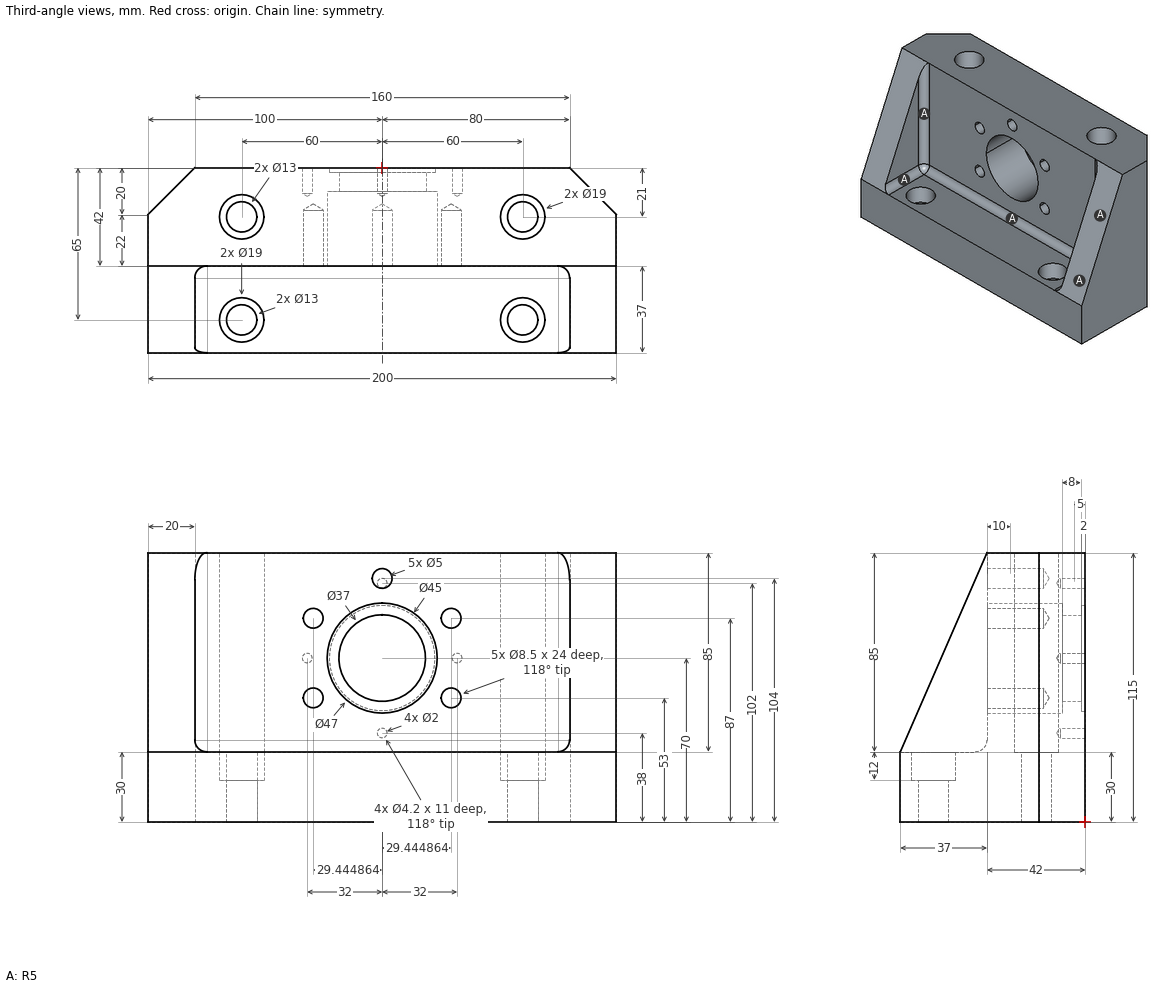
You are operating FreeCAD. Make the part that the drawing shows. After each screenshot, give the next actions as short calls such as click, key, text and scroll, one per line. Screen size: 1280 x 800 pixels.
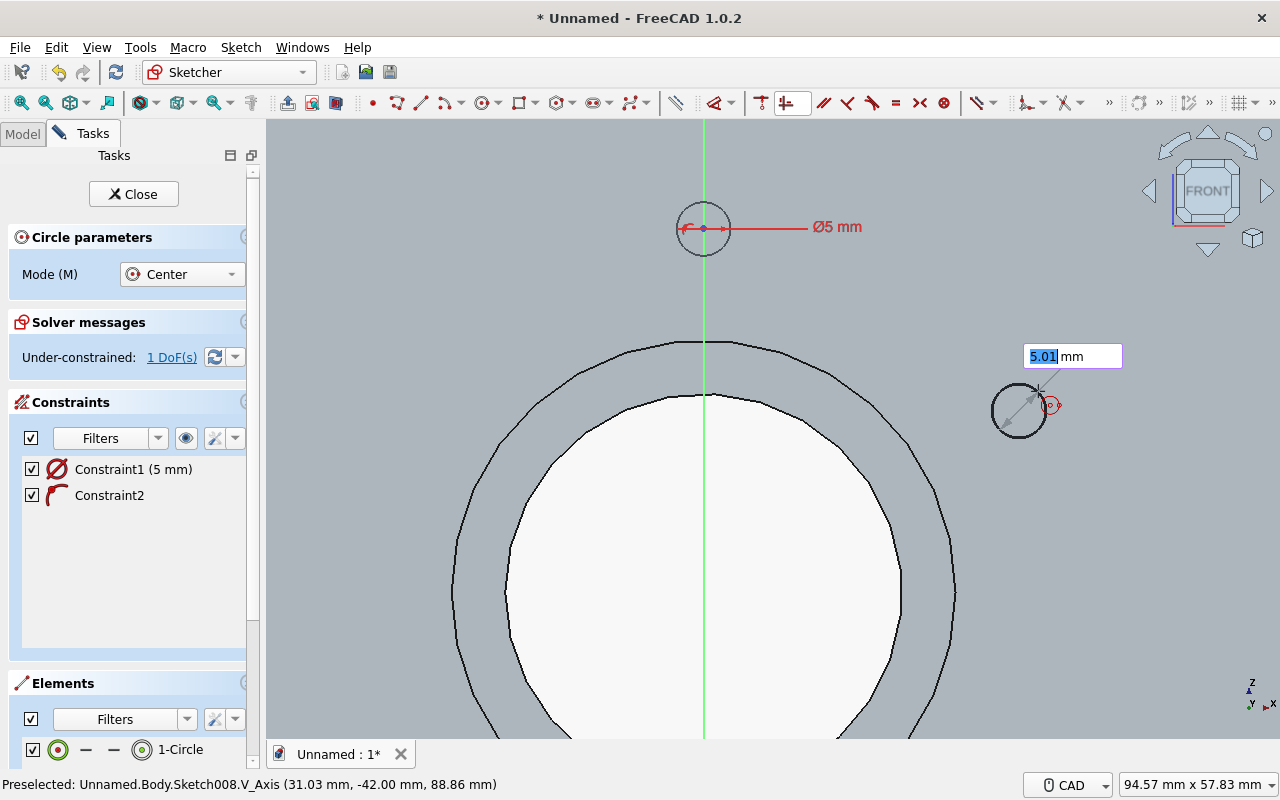
text(5)
key(Return)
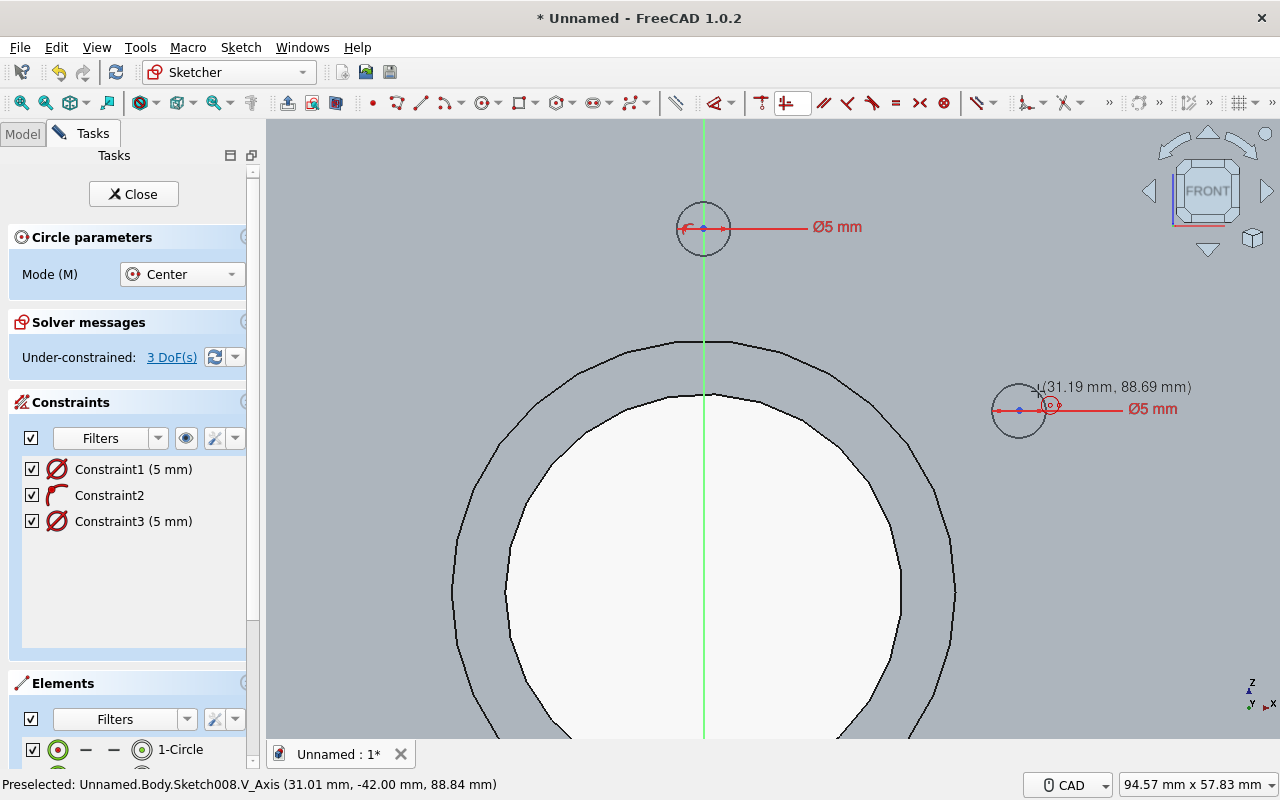
scroll(705, 229, down, 5)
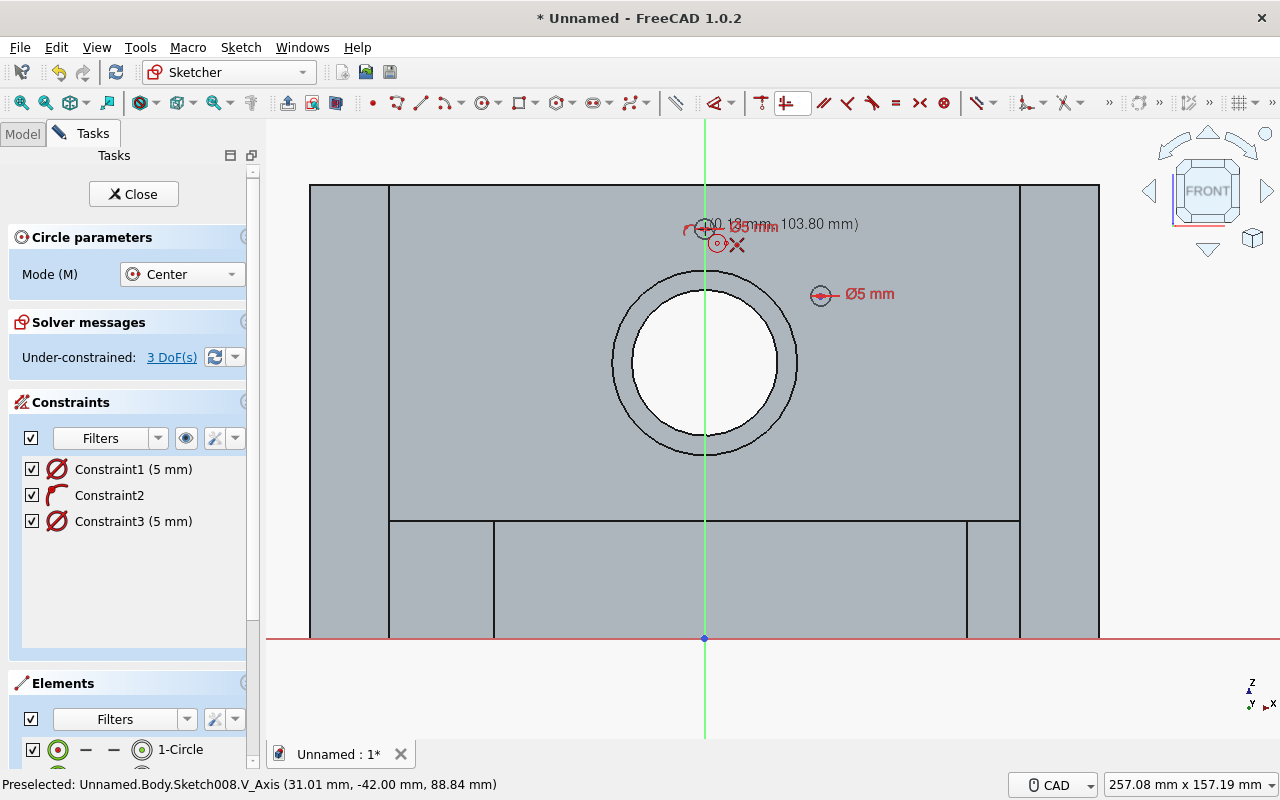
scroll(821, 430, up, 5)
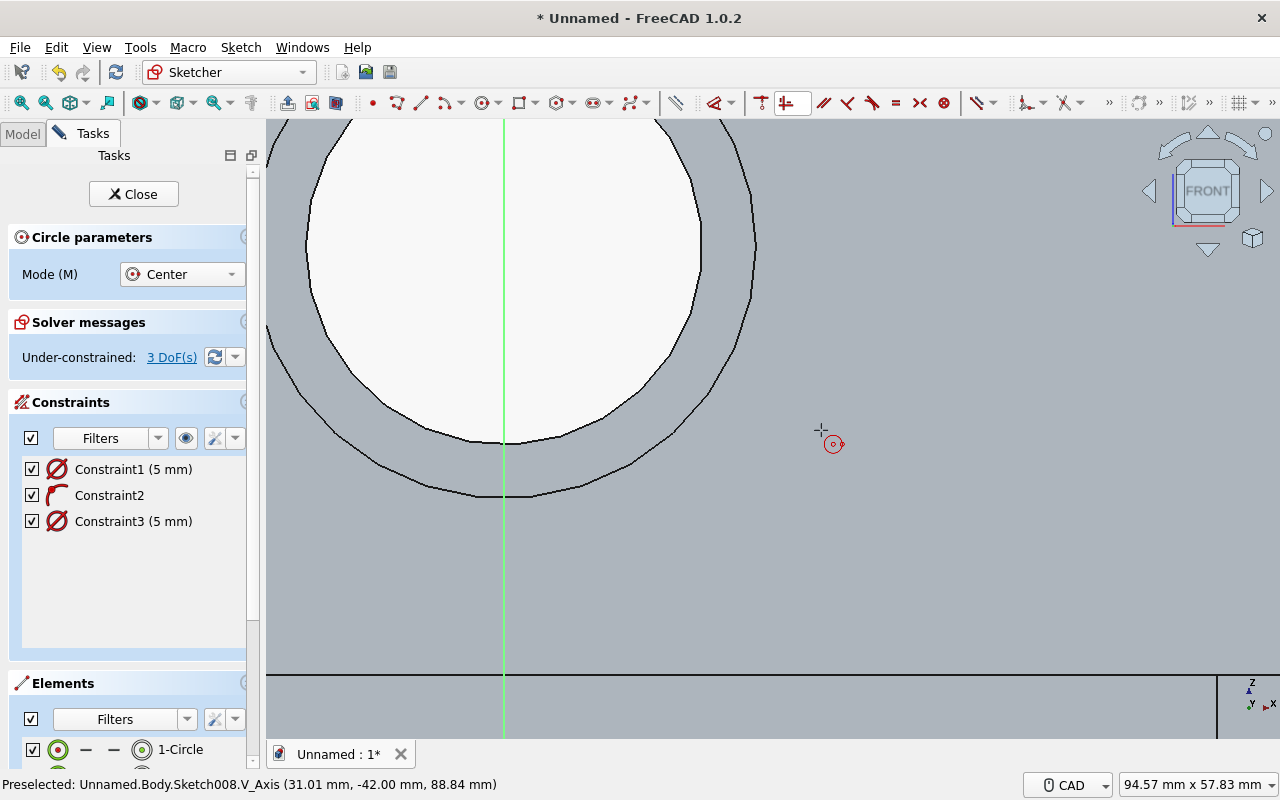
click(820, 429)
move(839, 410)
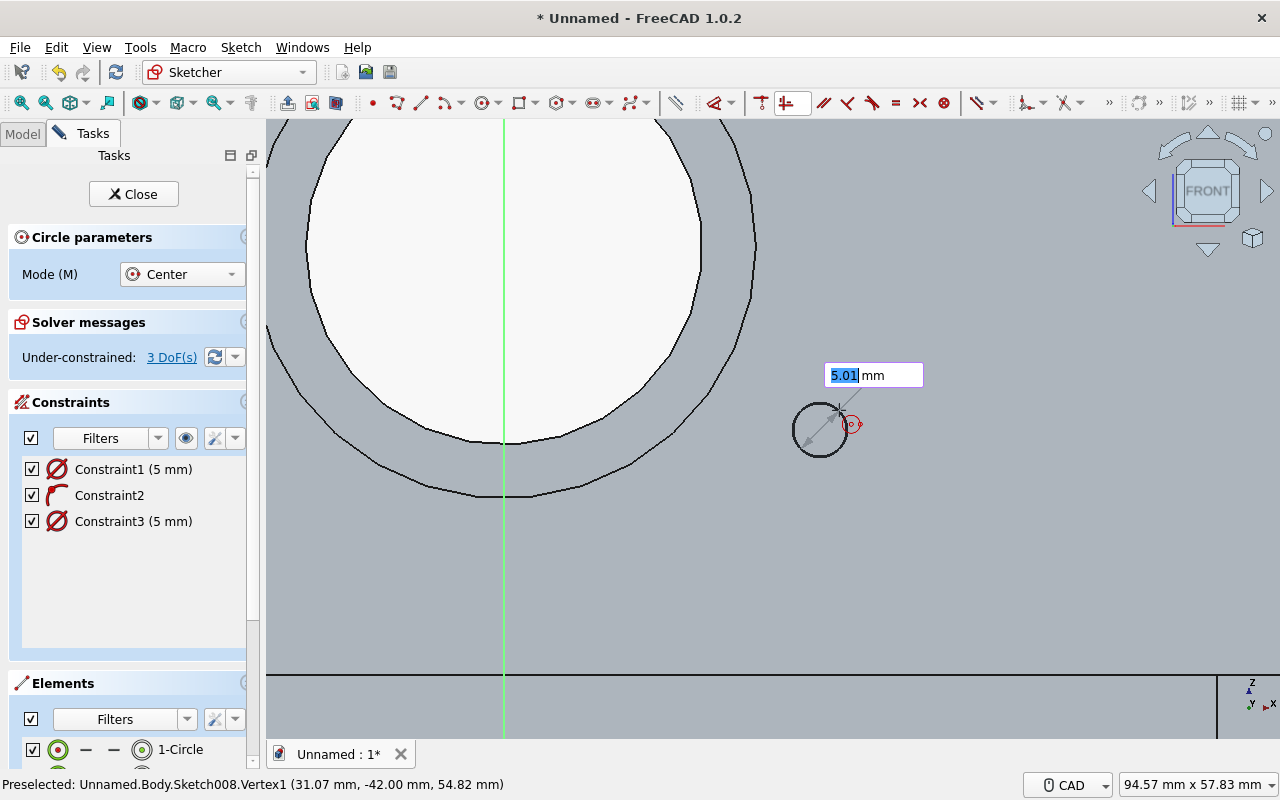
text(5)
key(Return)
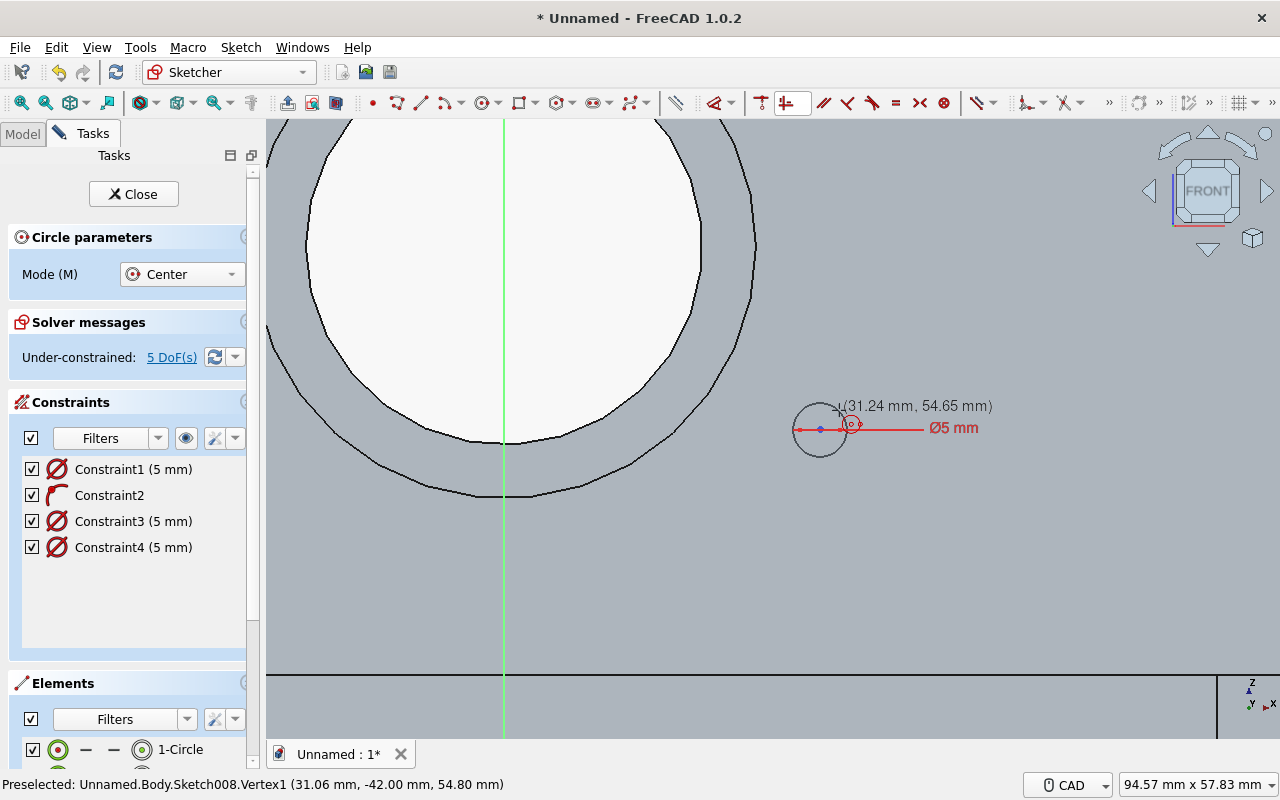
scroll(821, 431, down, 5)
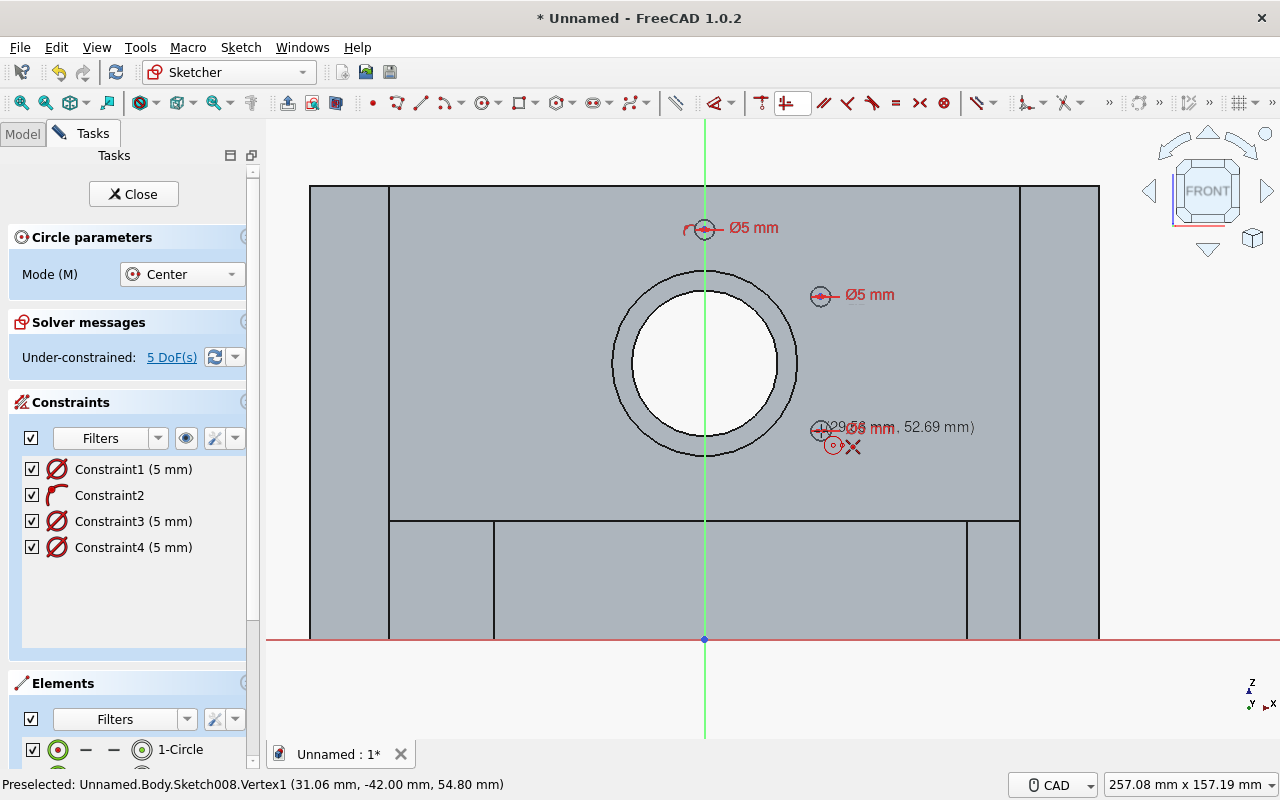
scroll(589, 296, up, 5)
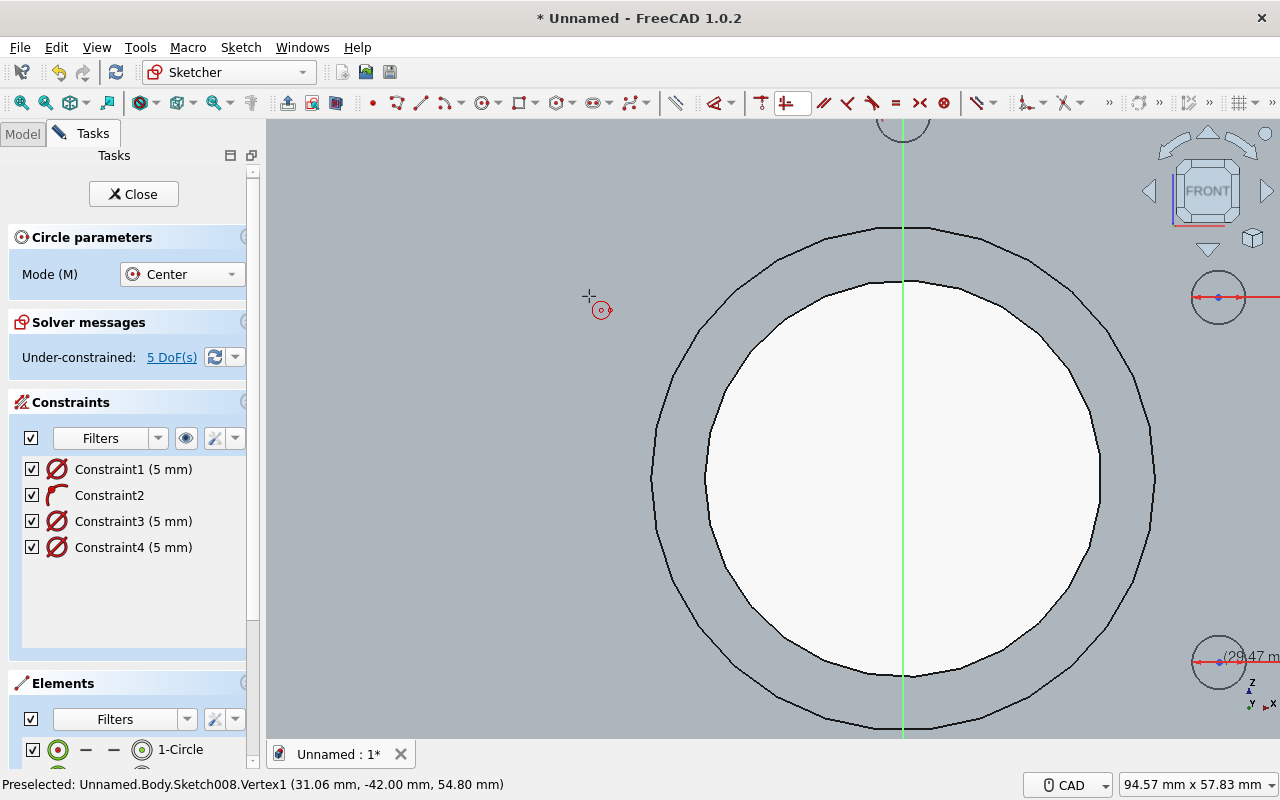
click(587, 296)
move(606, 278)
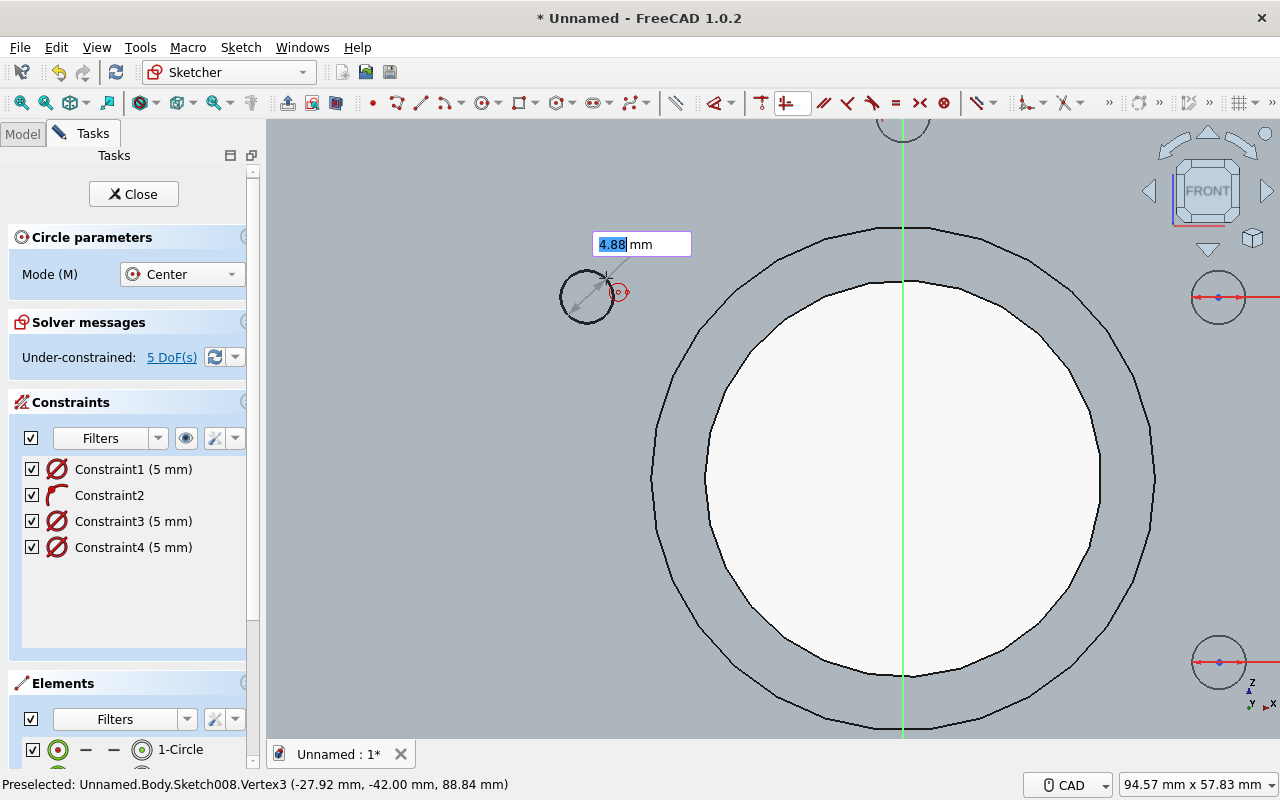
text(5)
key(Return)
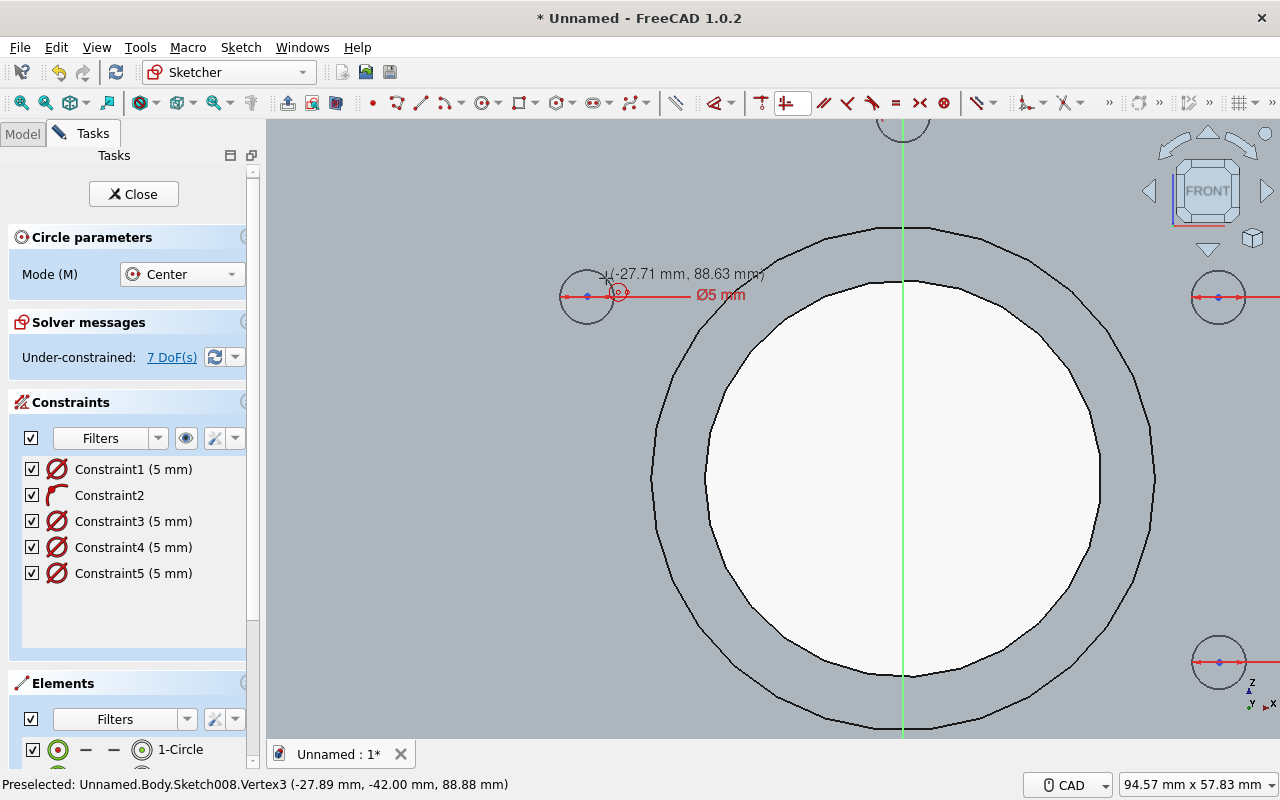
click(587, 661)
move(606, 642)